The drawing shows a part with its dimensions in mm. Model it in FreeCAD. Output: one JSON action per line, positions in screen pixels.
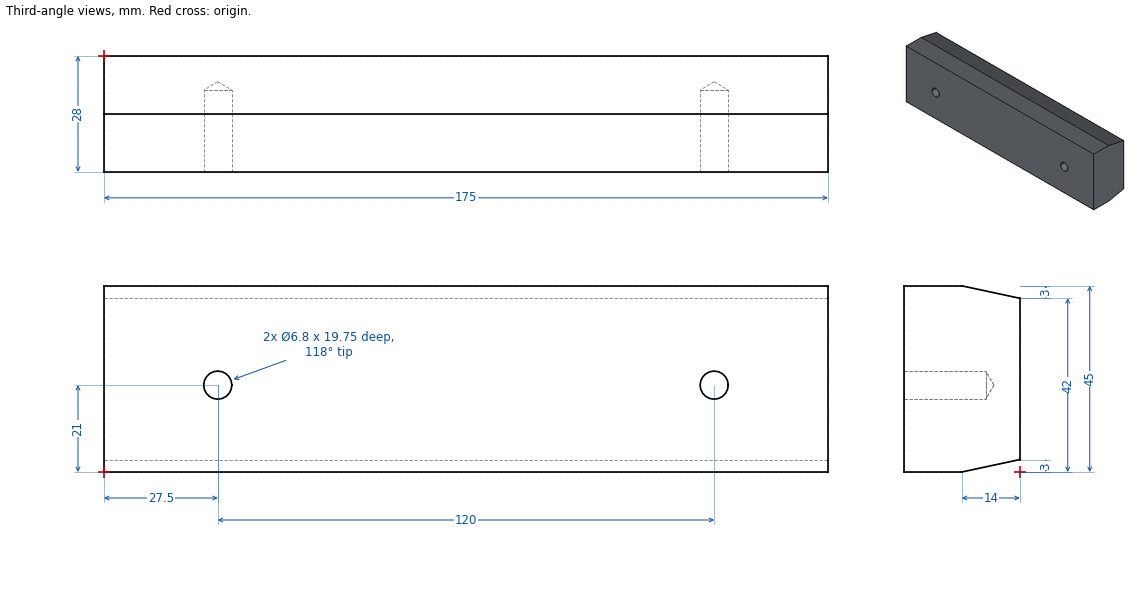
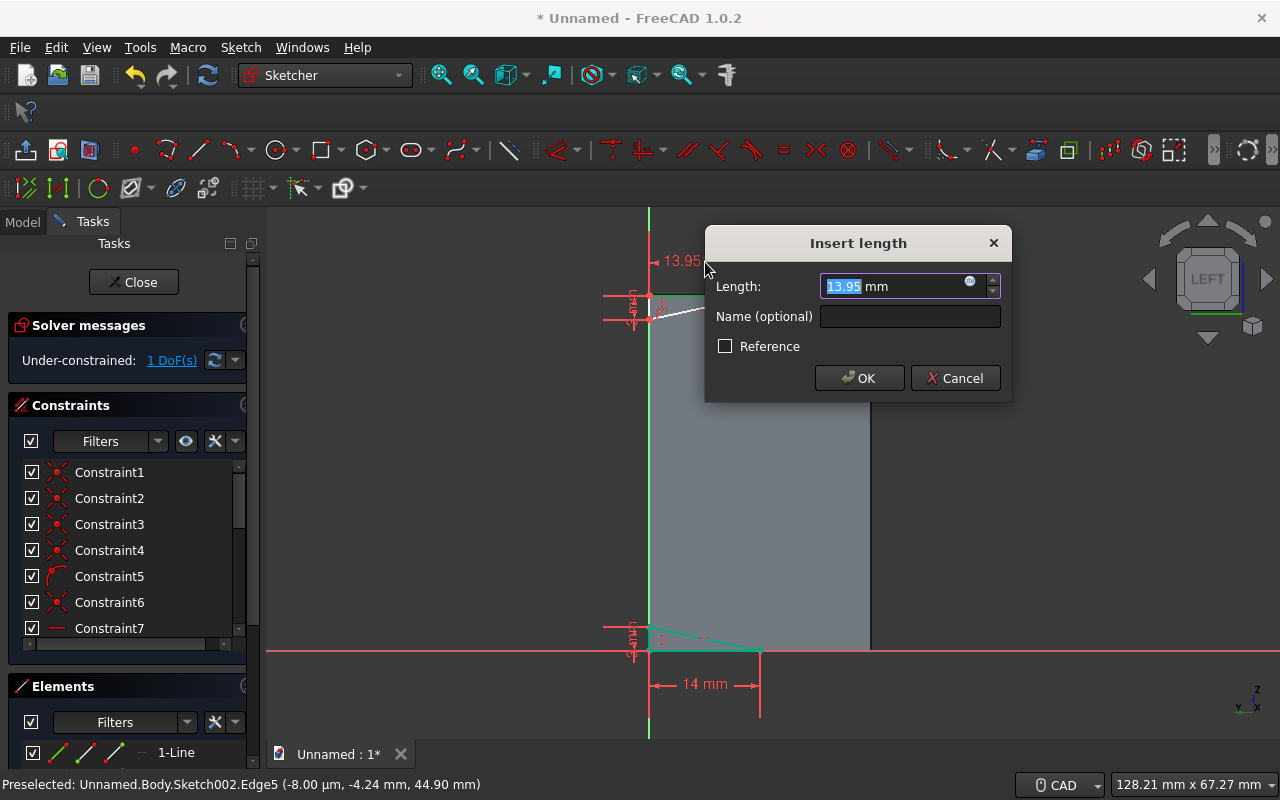
{"action": "type", "text": "14"}
{"action": "key", "text": "Return"}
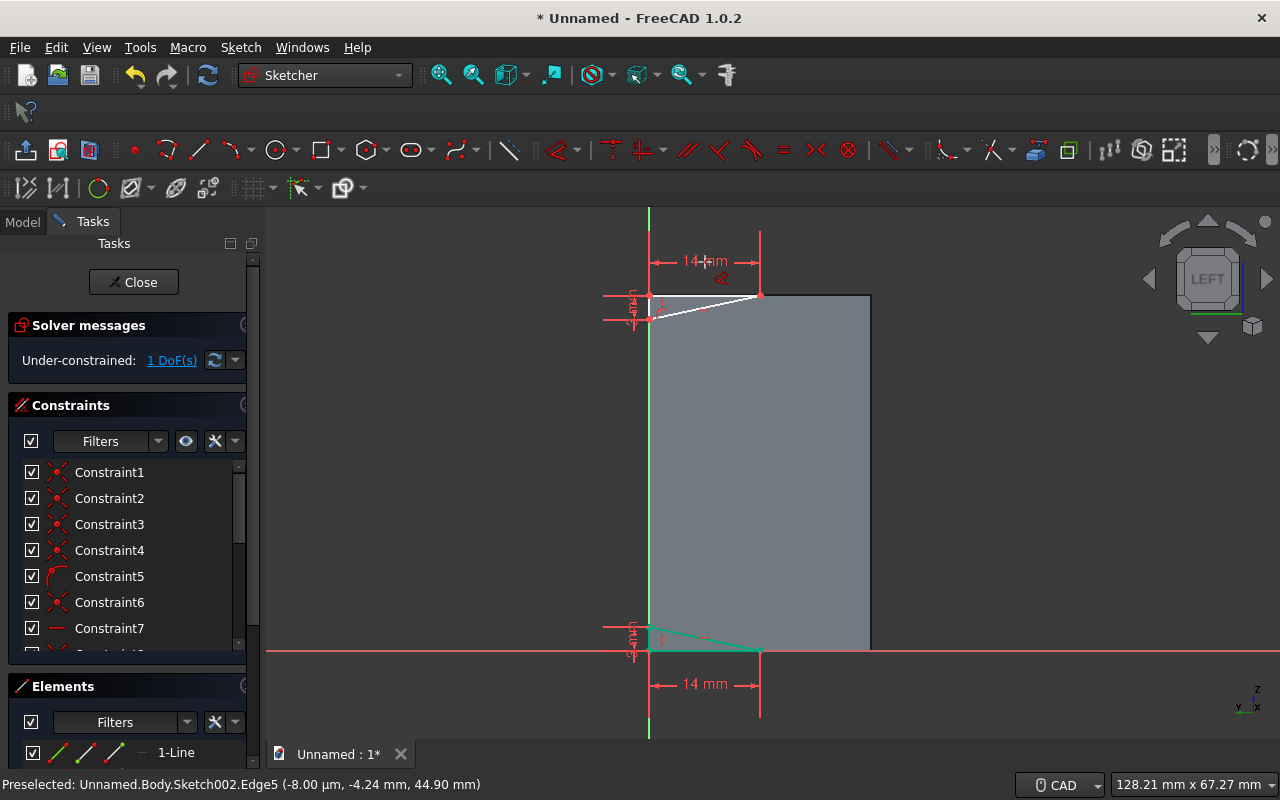
{"action": "left_click", "coordinate": [649, 320]}
{"action": "left_click", "coordinate": [615, 485]}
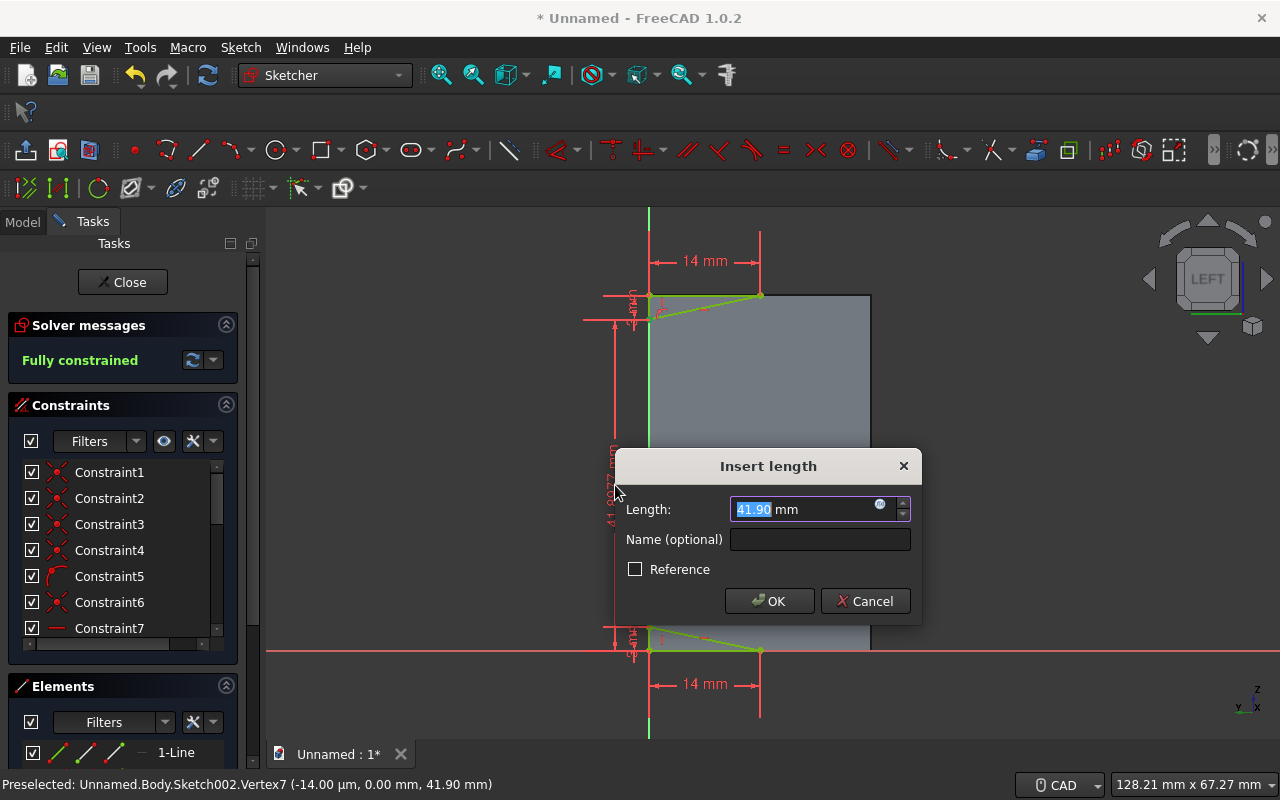
{"action": "type", "text": "42"}
{"action": "key", "text": "Return"}
{"action": "key", "text": "Escape"}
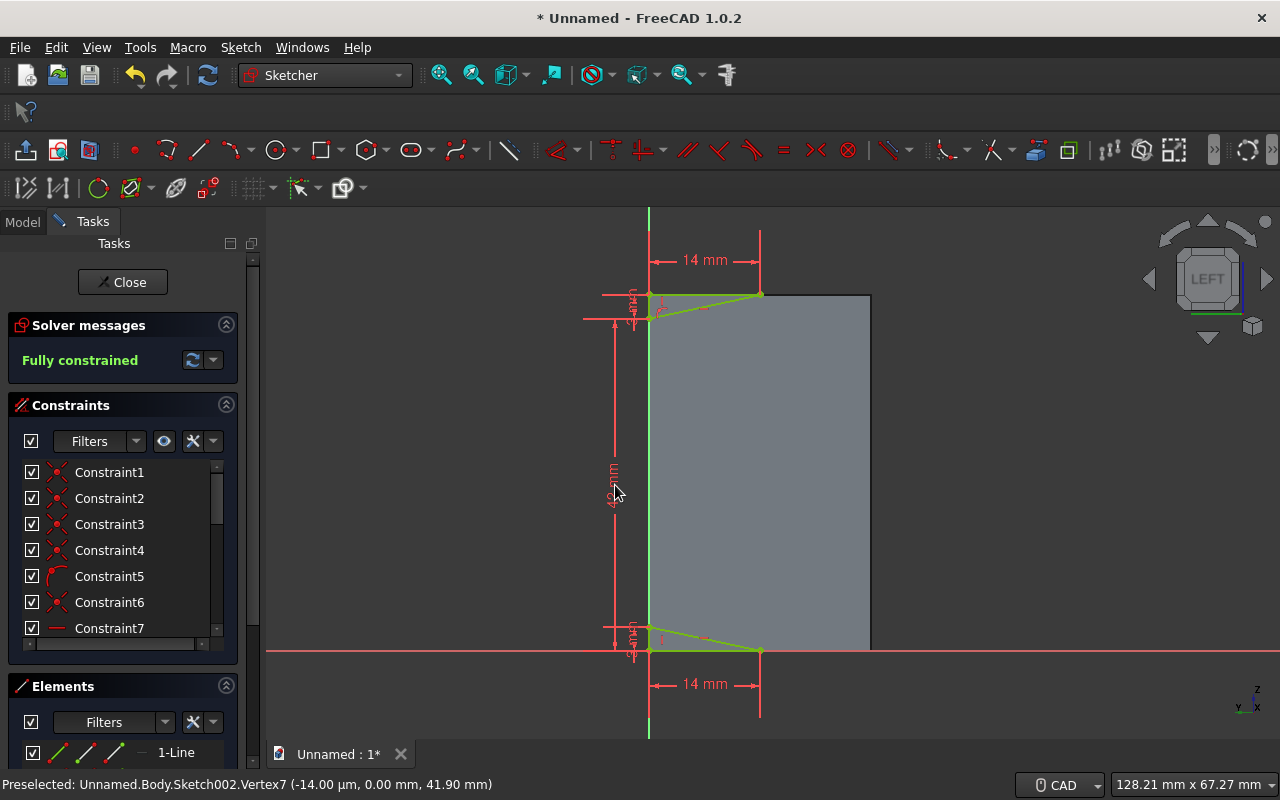
{"action": "left_click", "coordinate": [123, 282]}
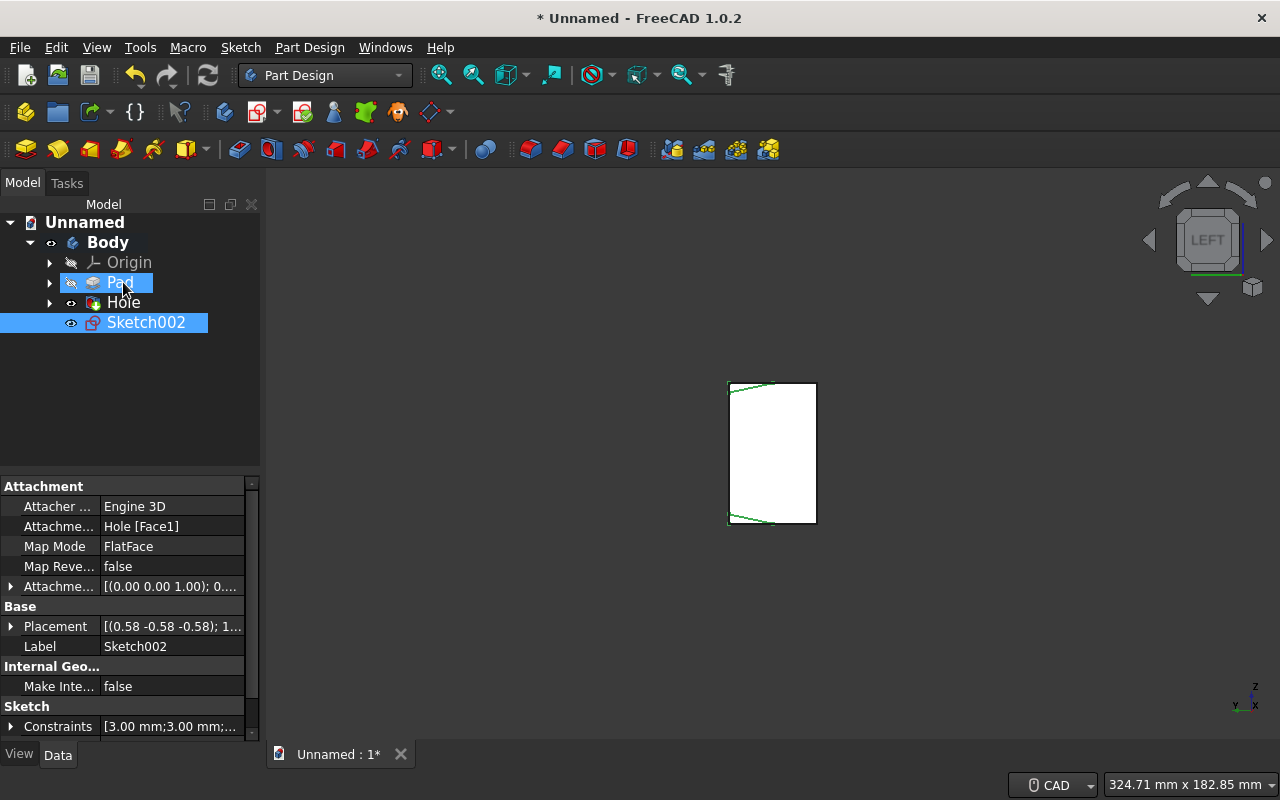
{"action": "left_click", "coordinate": [240, 150]}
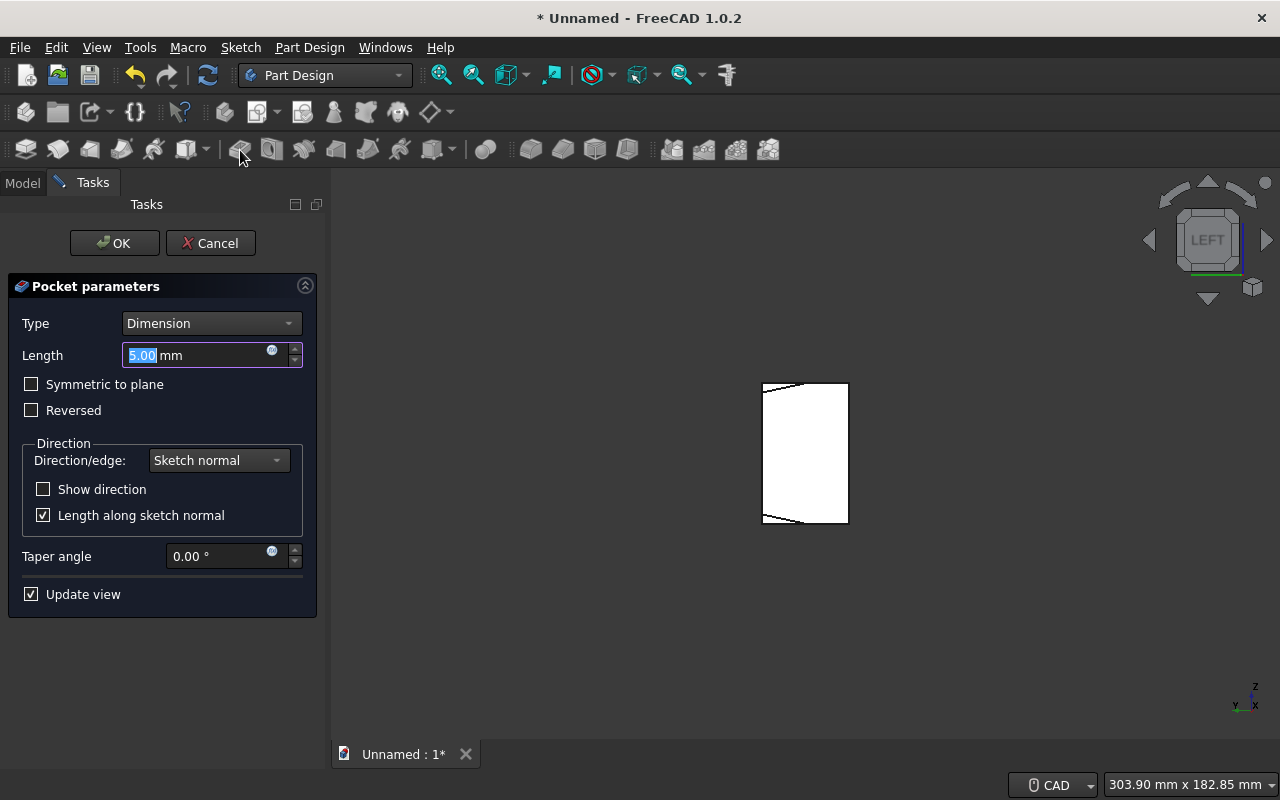
{"action": "left_click", "coordinate": [212, 324]}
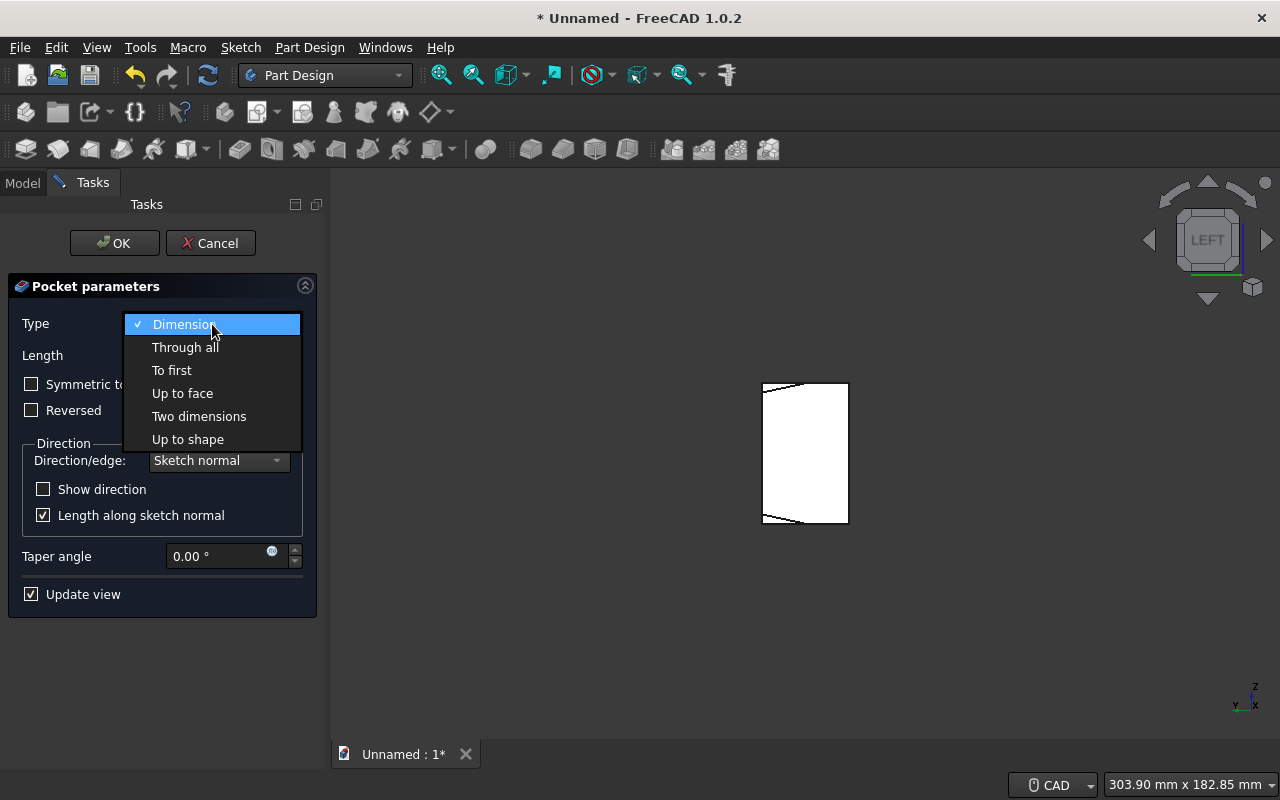
{"action": "left_click", "coordinate": [212, 348]}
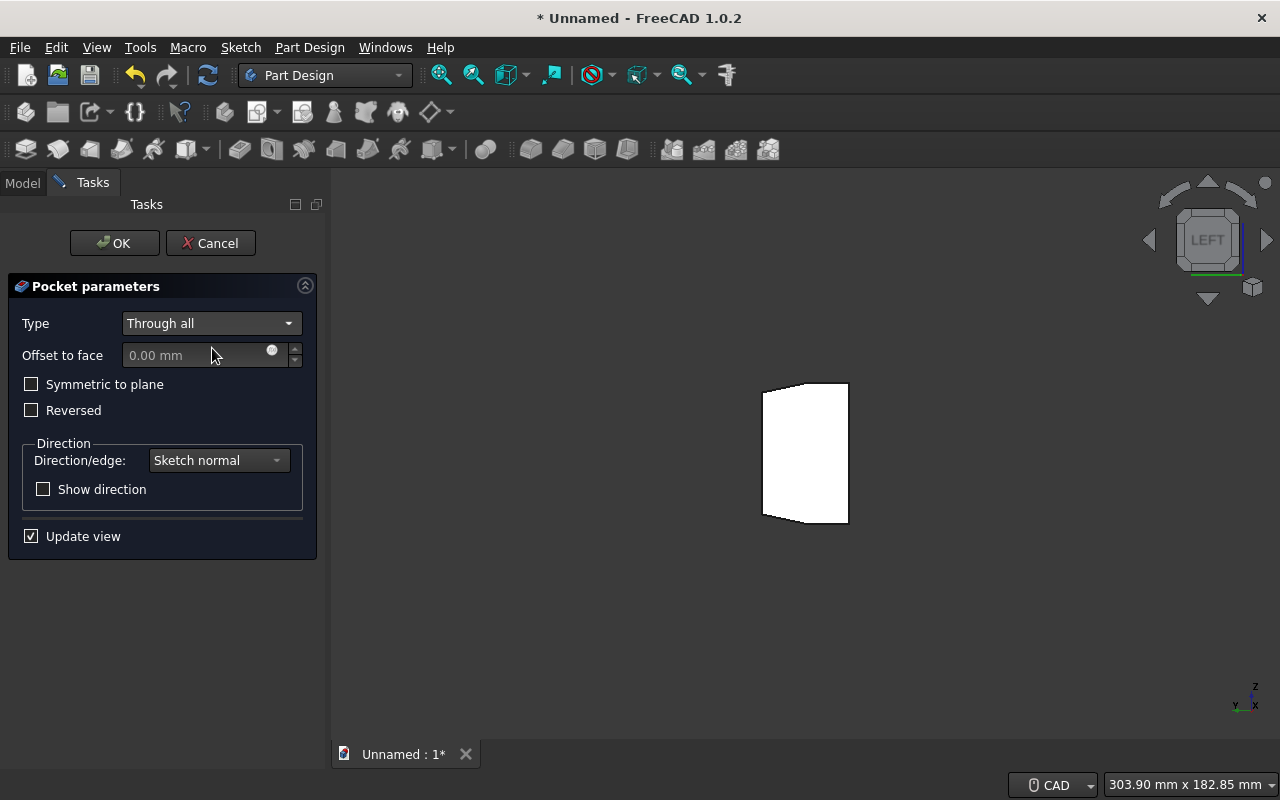
{"action": "left_click", "coordinate": [115, 243]}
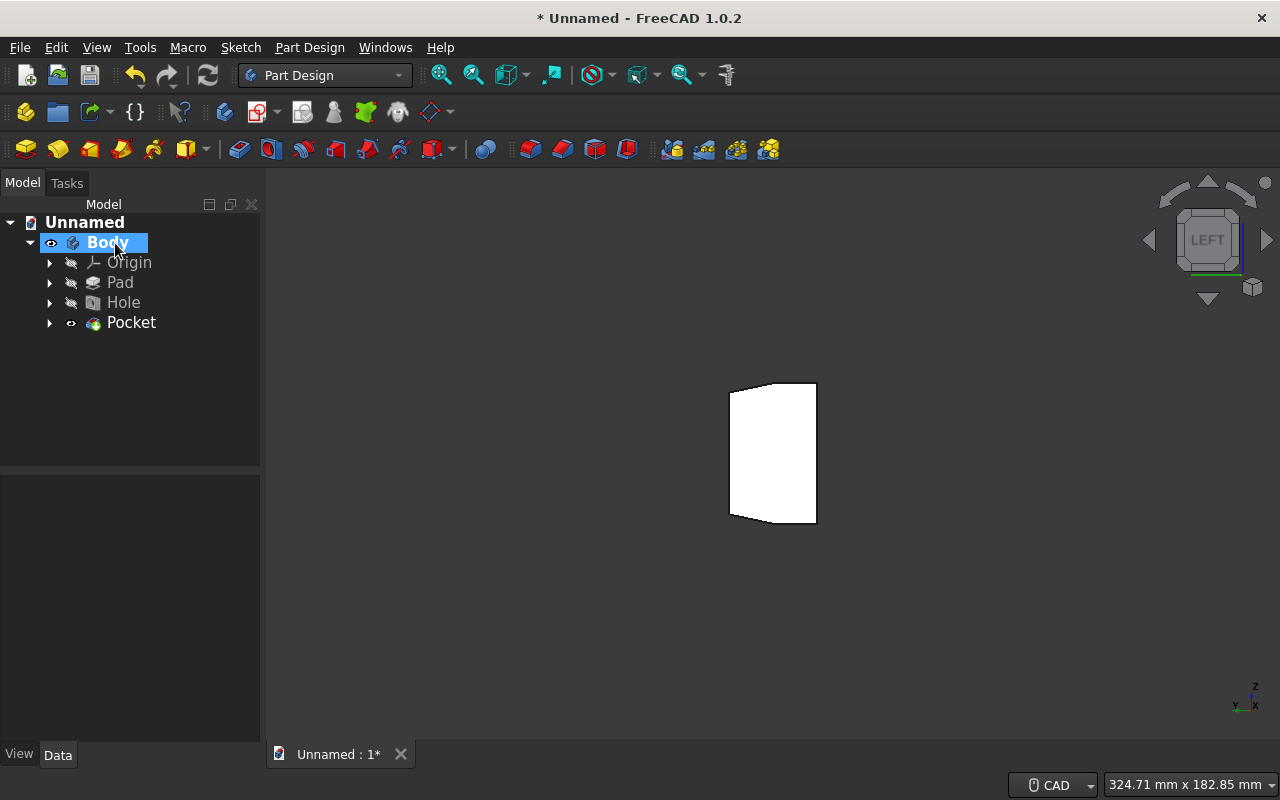
{"action": "key", "text": "0"}